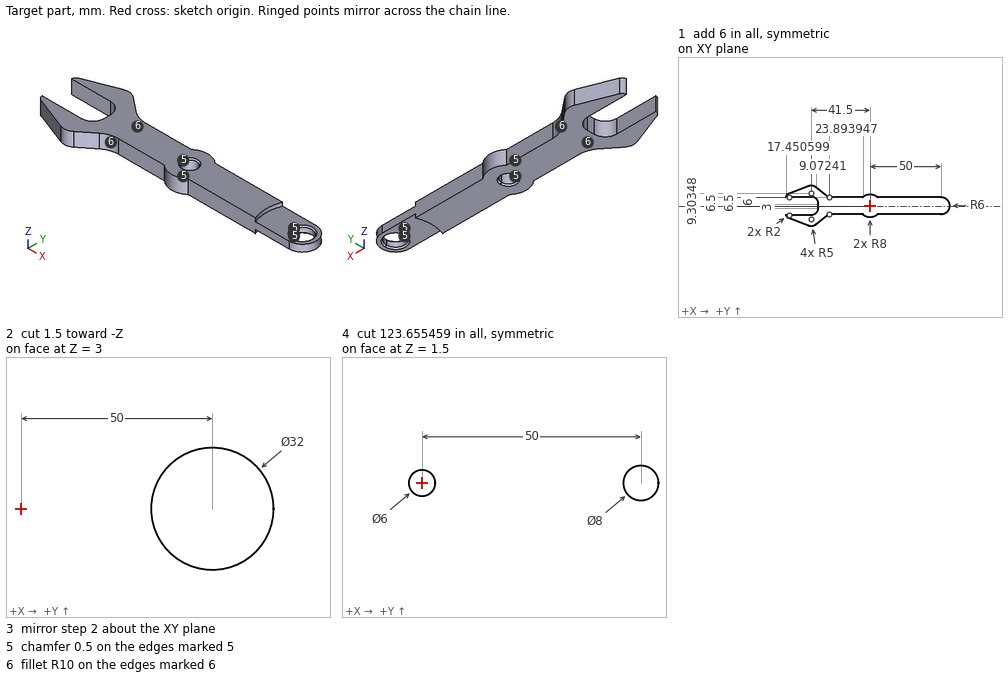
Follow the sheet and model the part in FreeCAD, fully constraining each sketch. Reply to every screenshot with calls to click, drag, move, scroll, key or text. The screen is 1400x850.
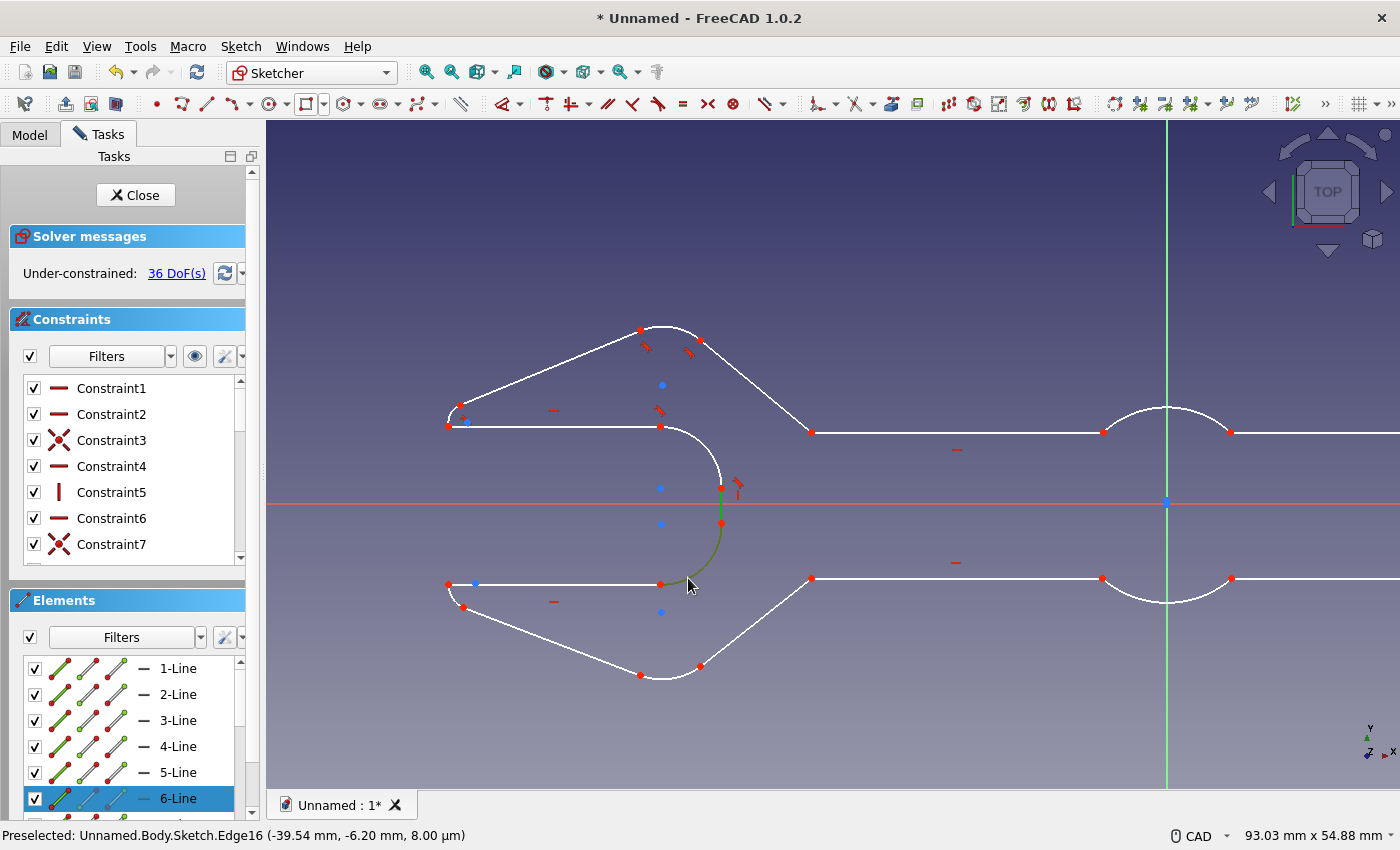
click(658, 104)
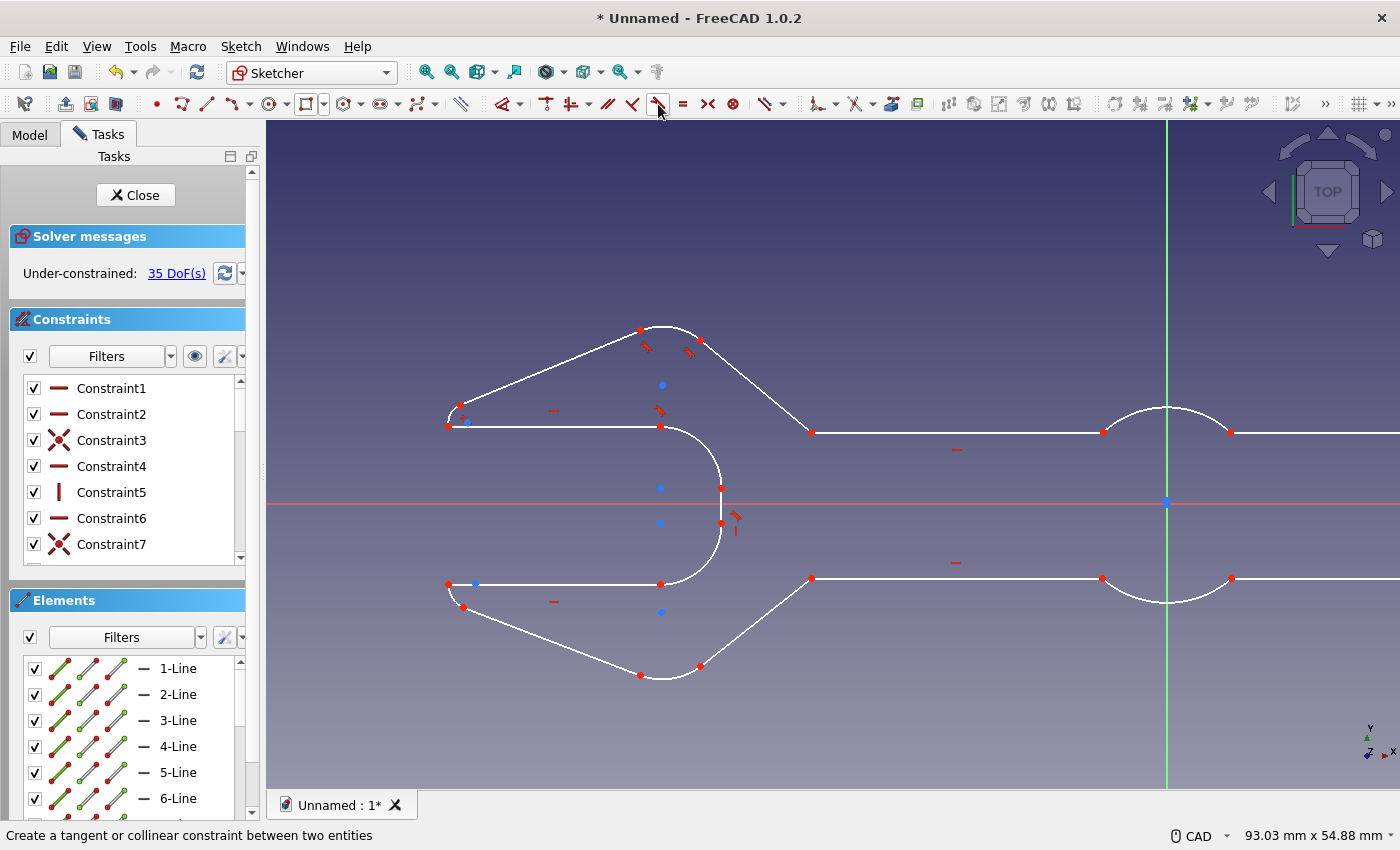
click(597, 585)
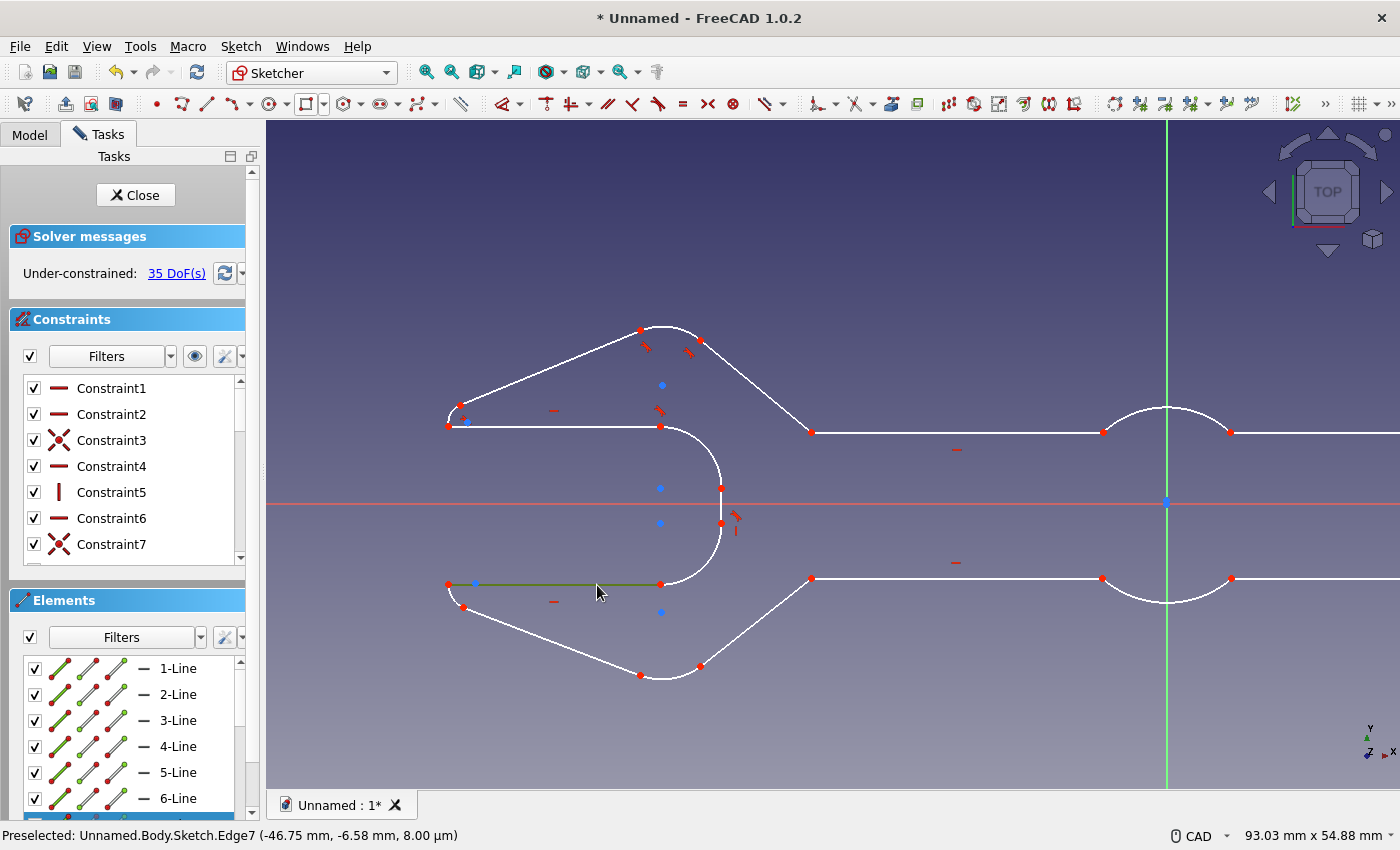
click(688, 578)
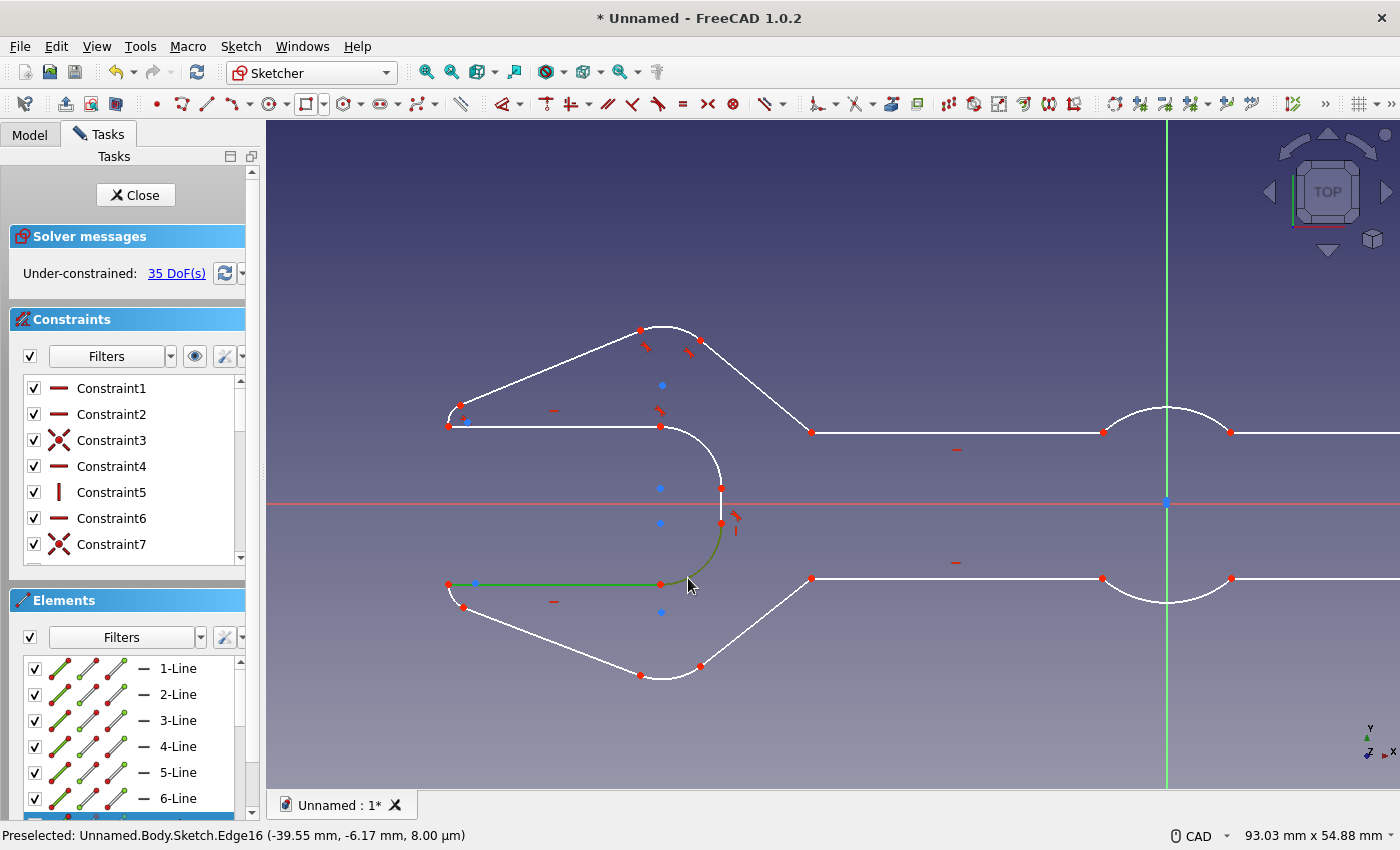
click(658, 104)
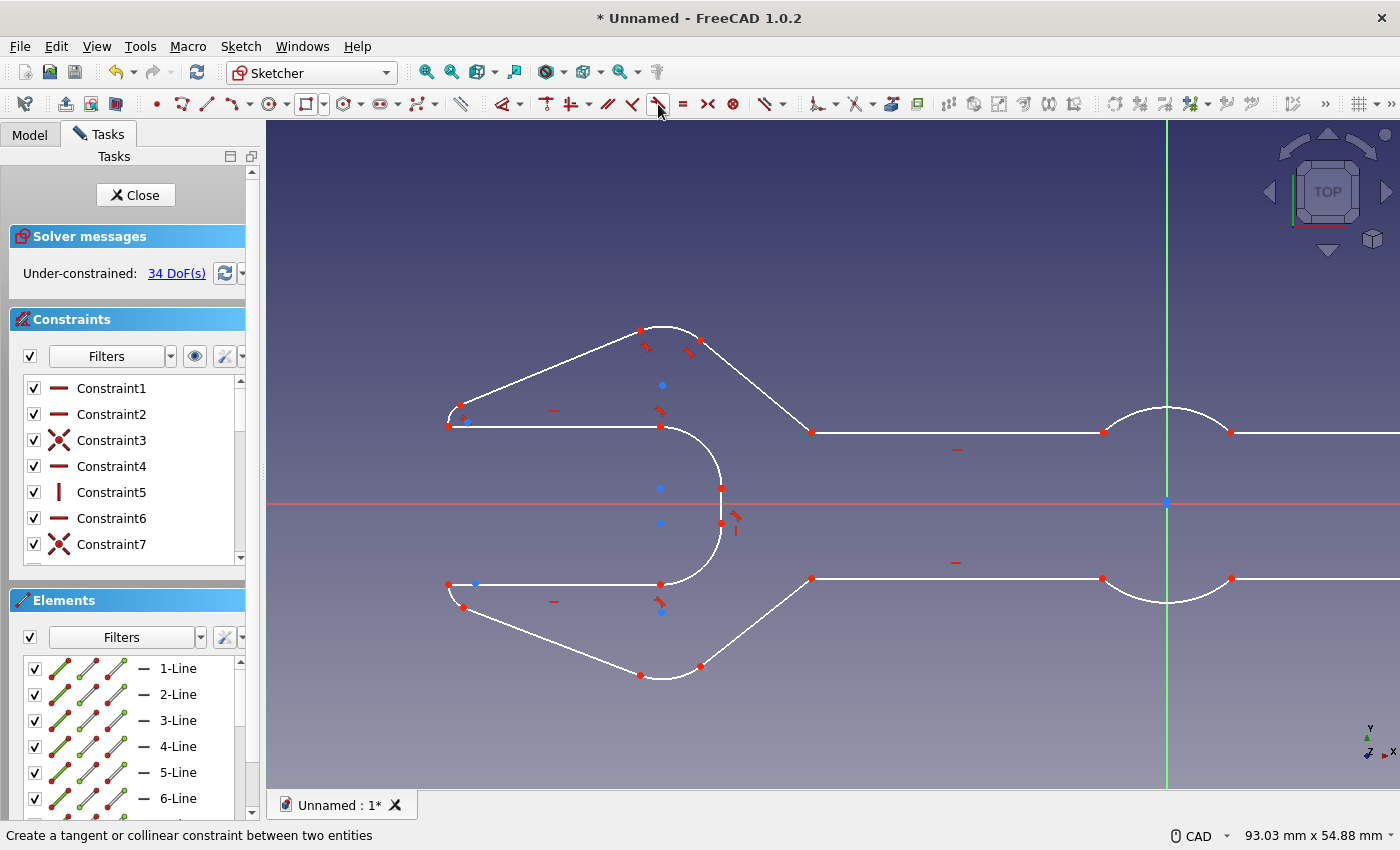
click(517, 628)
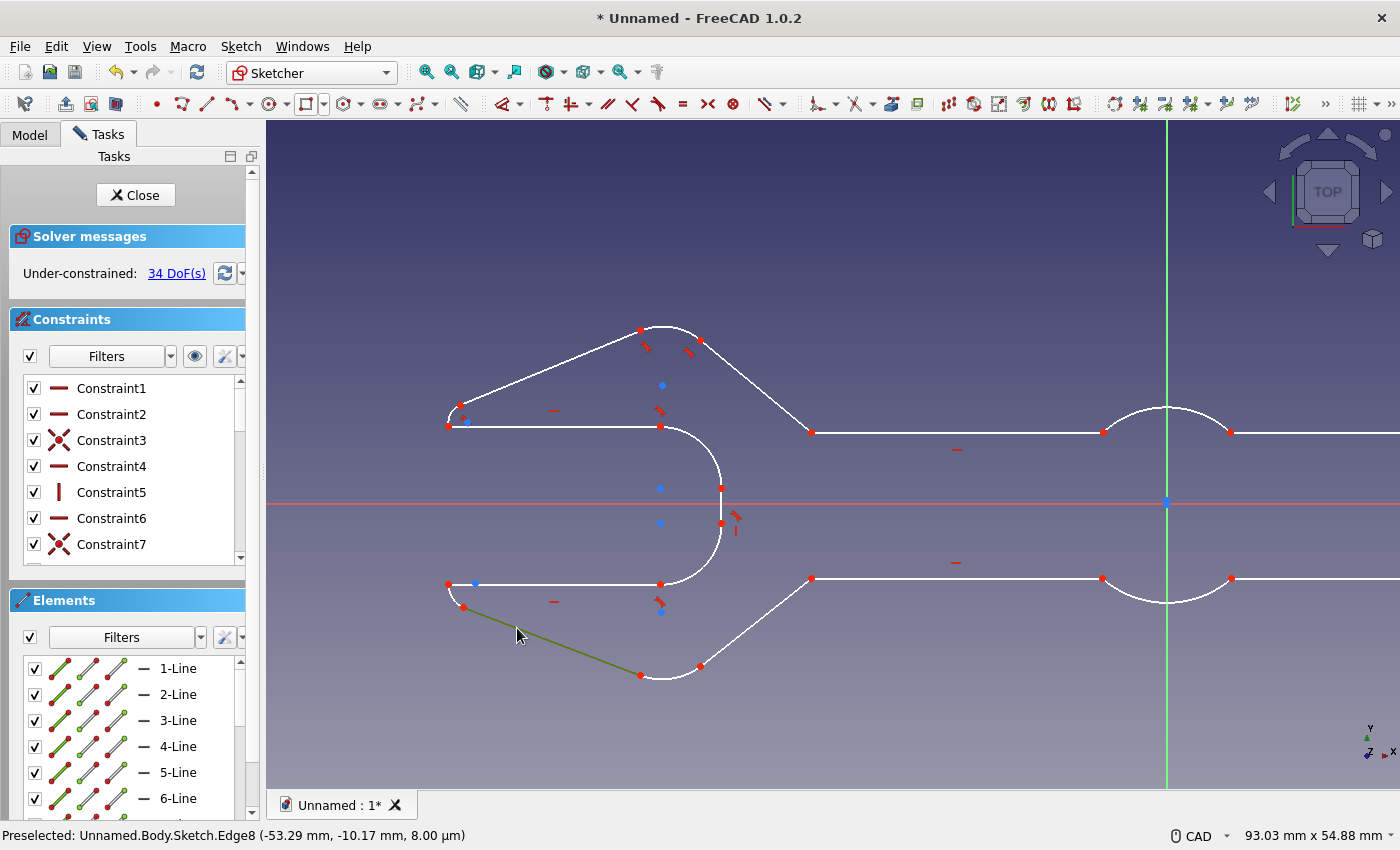
click(453, 598)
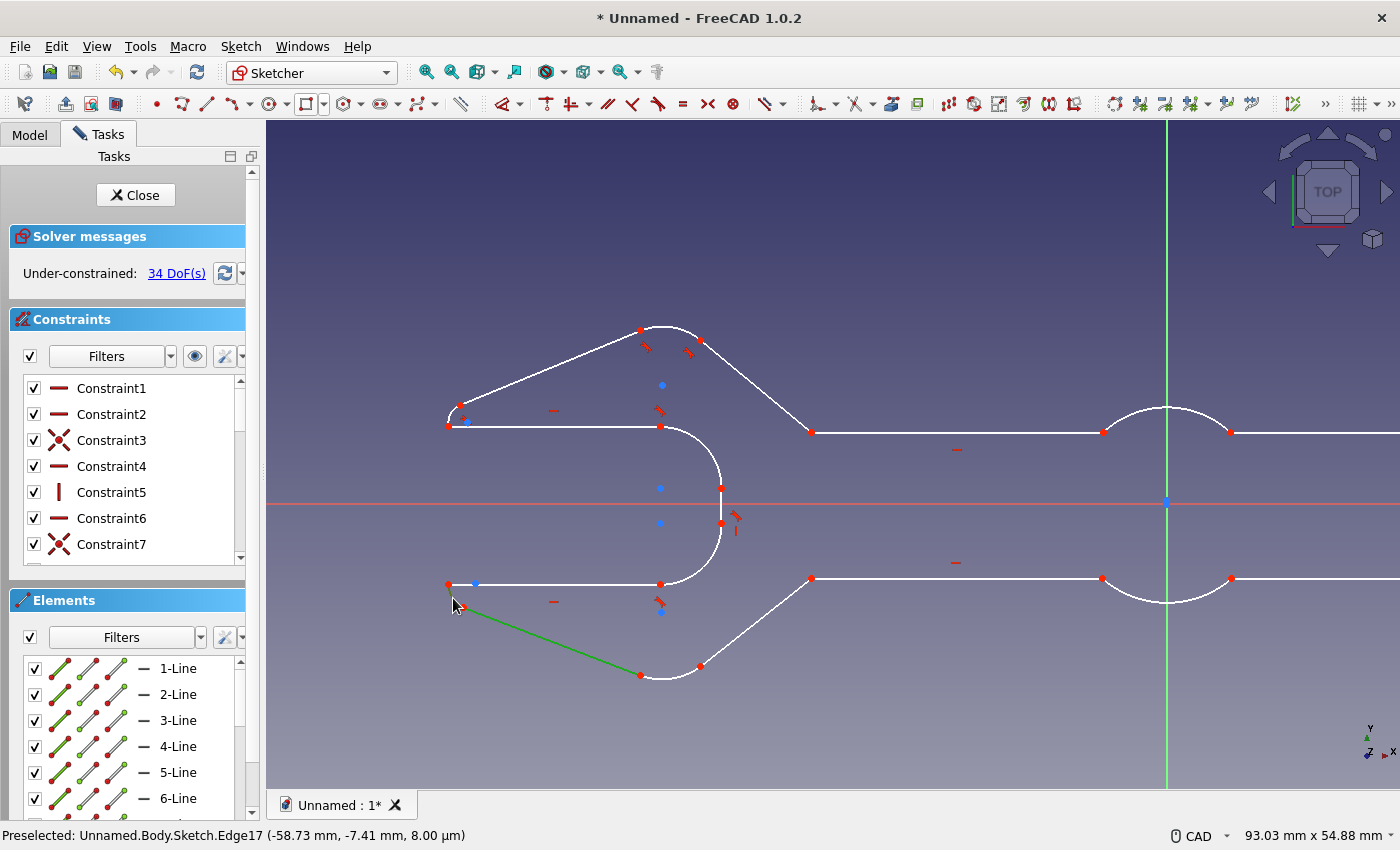
click(658, 104)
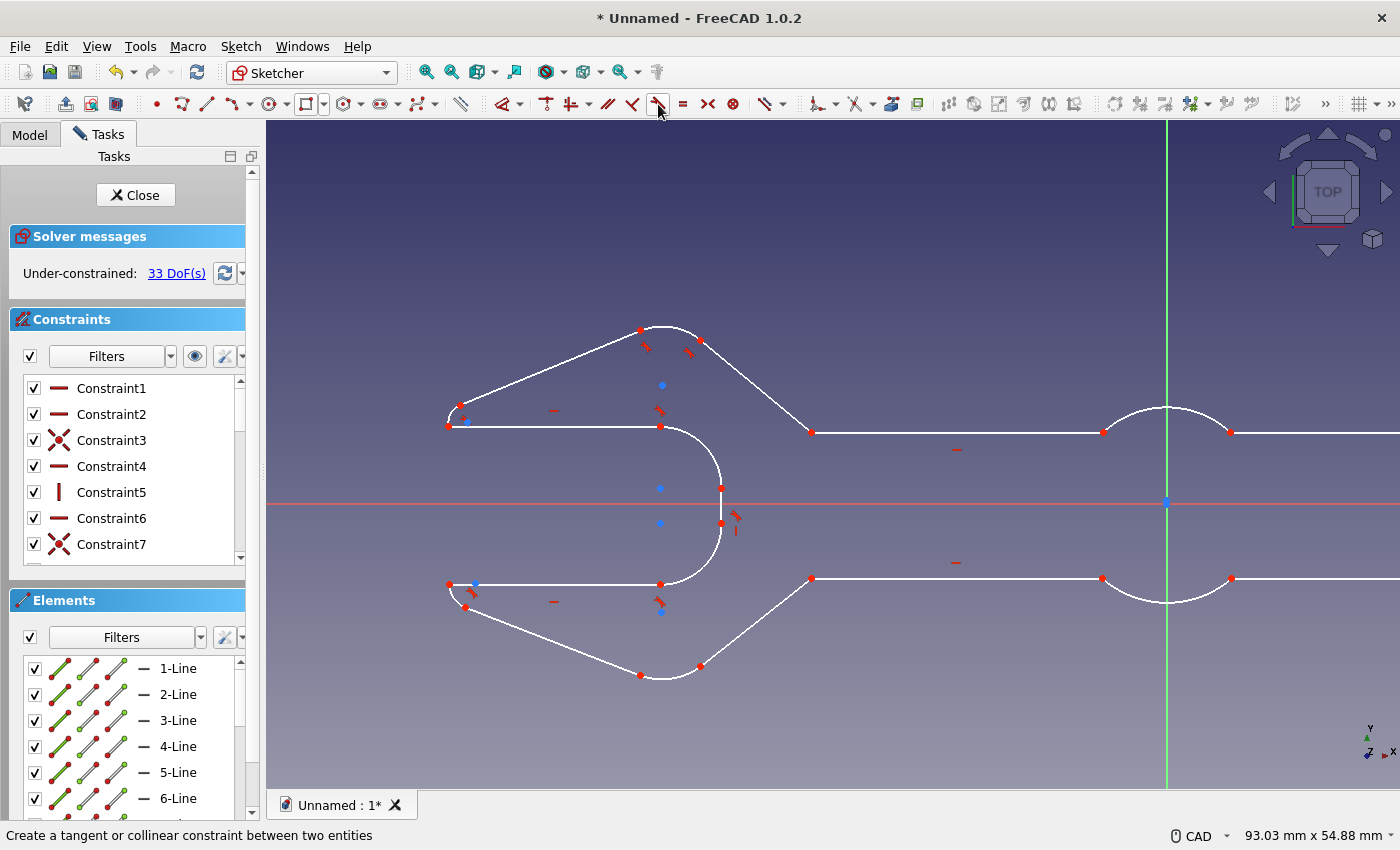
click(518, 628)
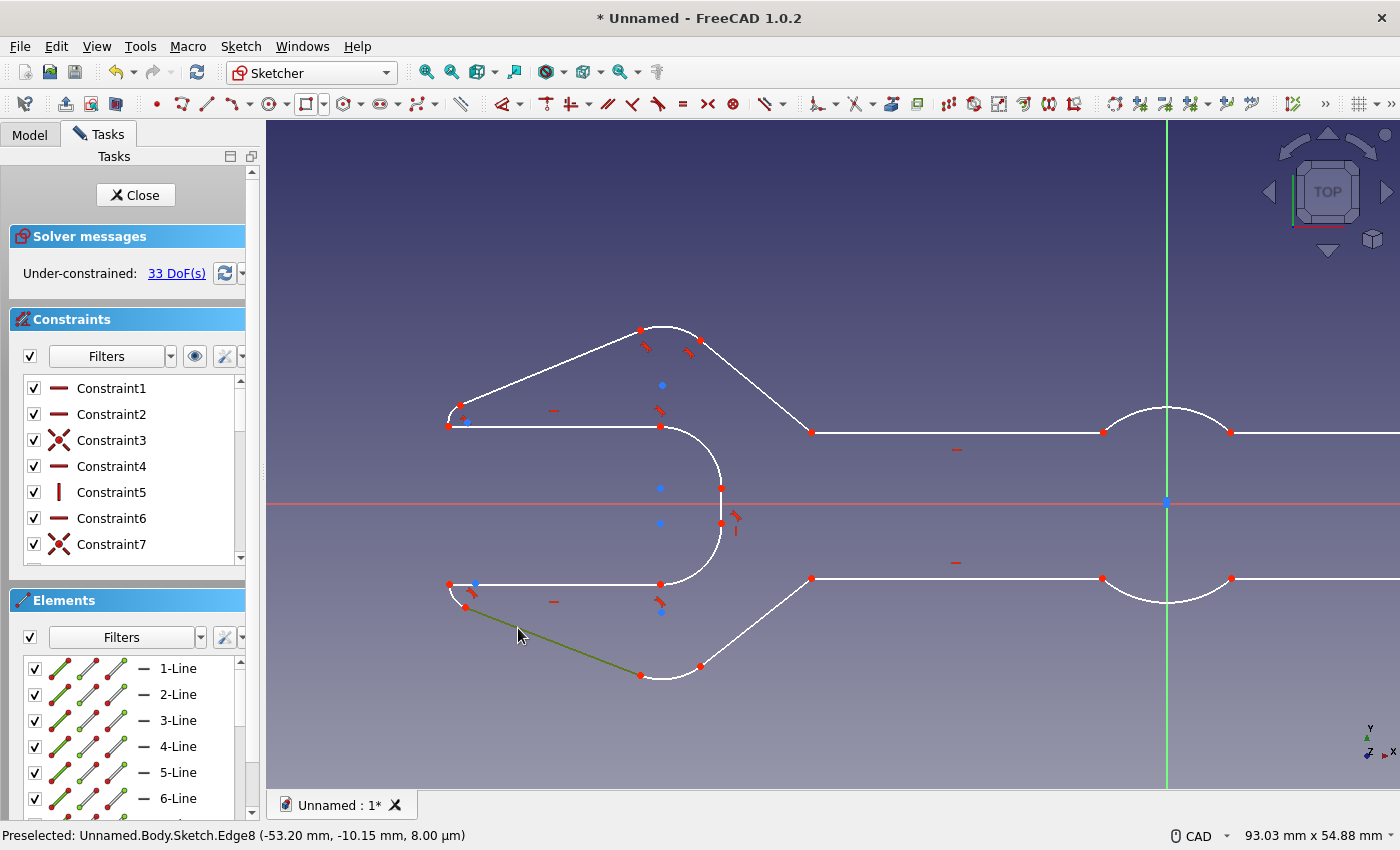
click(659, 679)